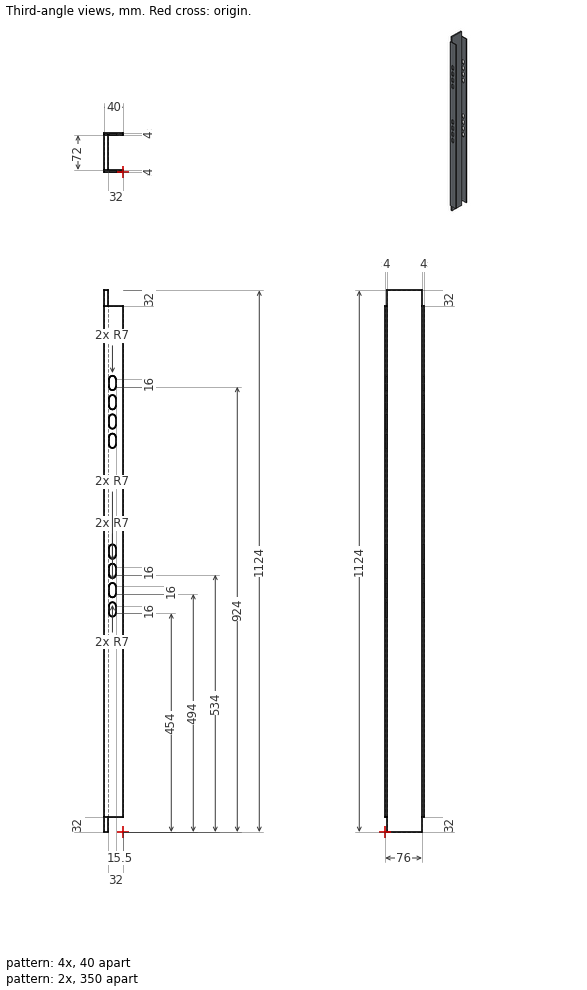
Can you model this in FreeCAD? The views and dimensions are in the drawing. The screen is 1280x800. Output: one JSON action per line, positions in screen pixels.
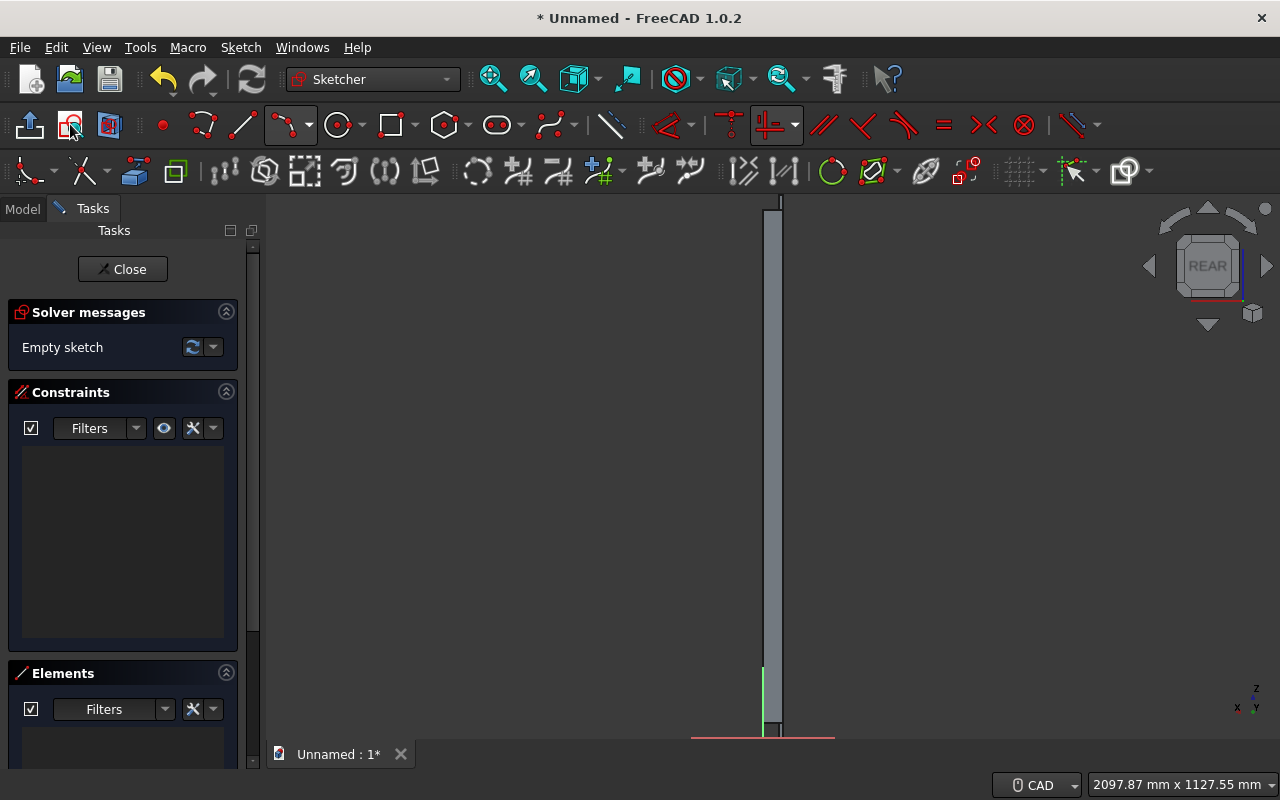
{"action": "scroll", "coordinate": [778, 278], "scroll_direction": "up", "scroll_amount": 15}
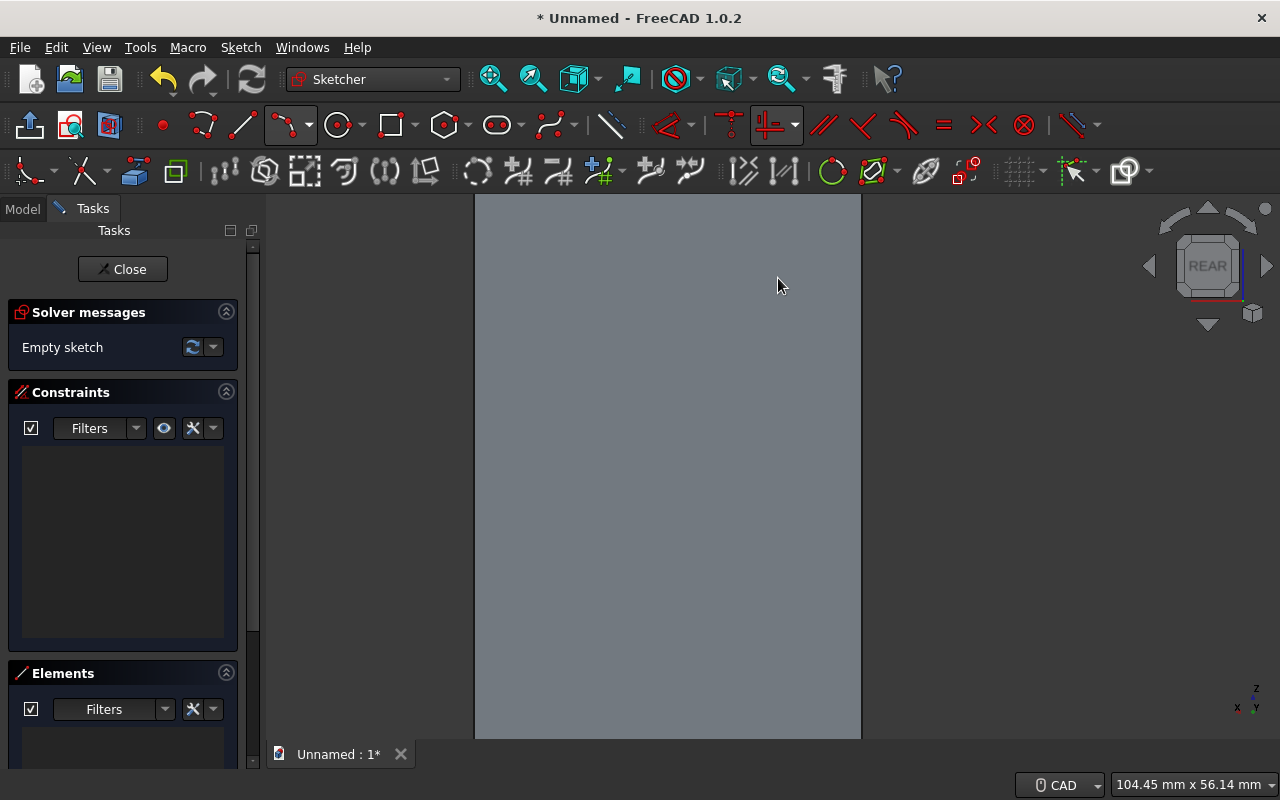
{"action": "left_click", "coordinate": [498, 126]}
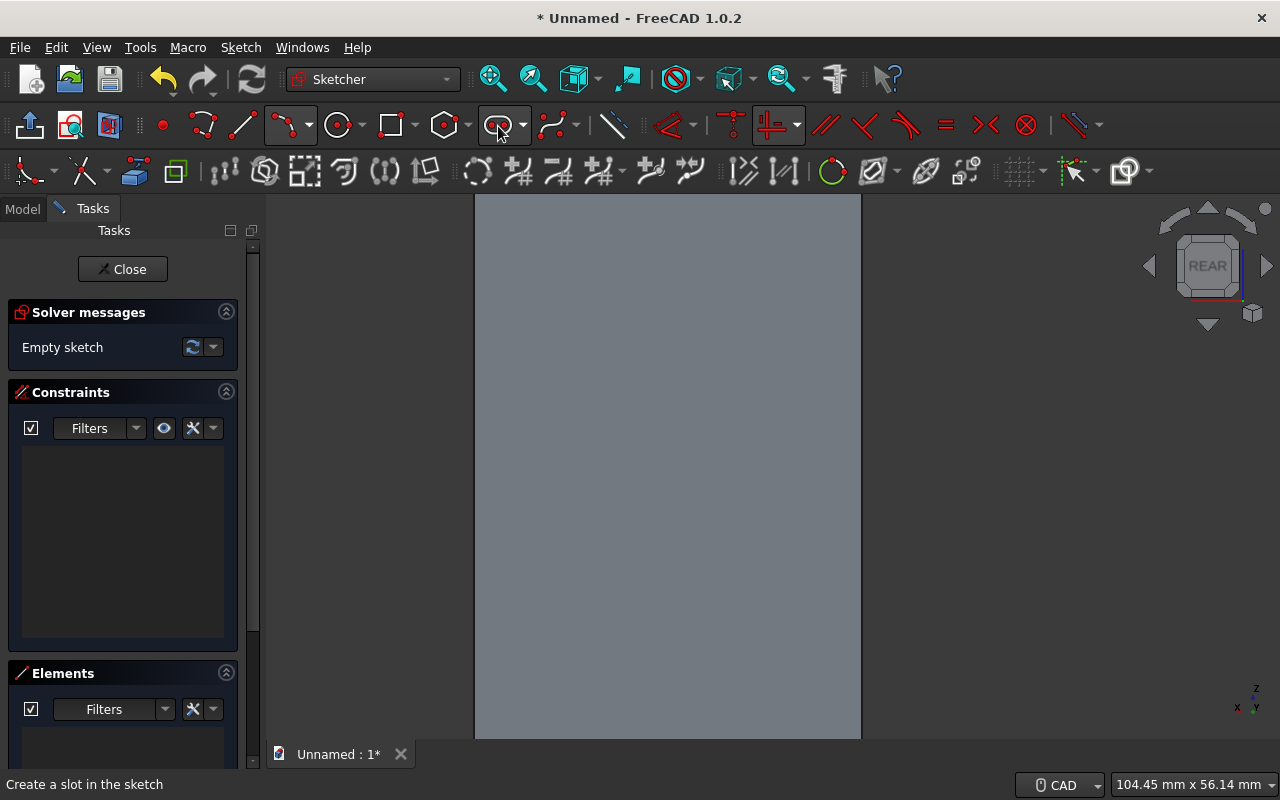
{"action": "left_click", "coordinate": [692, 547]}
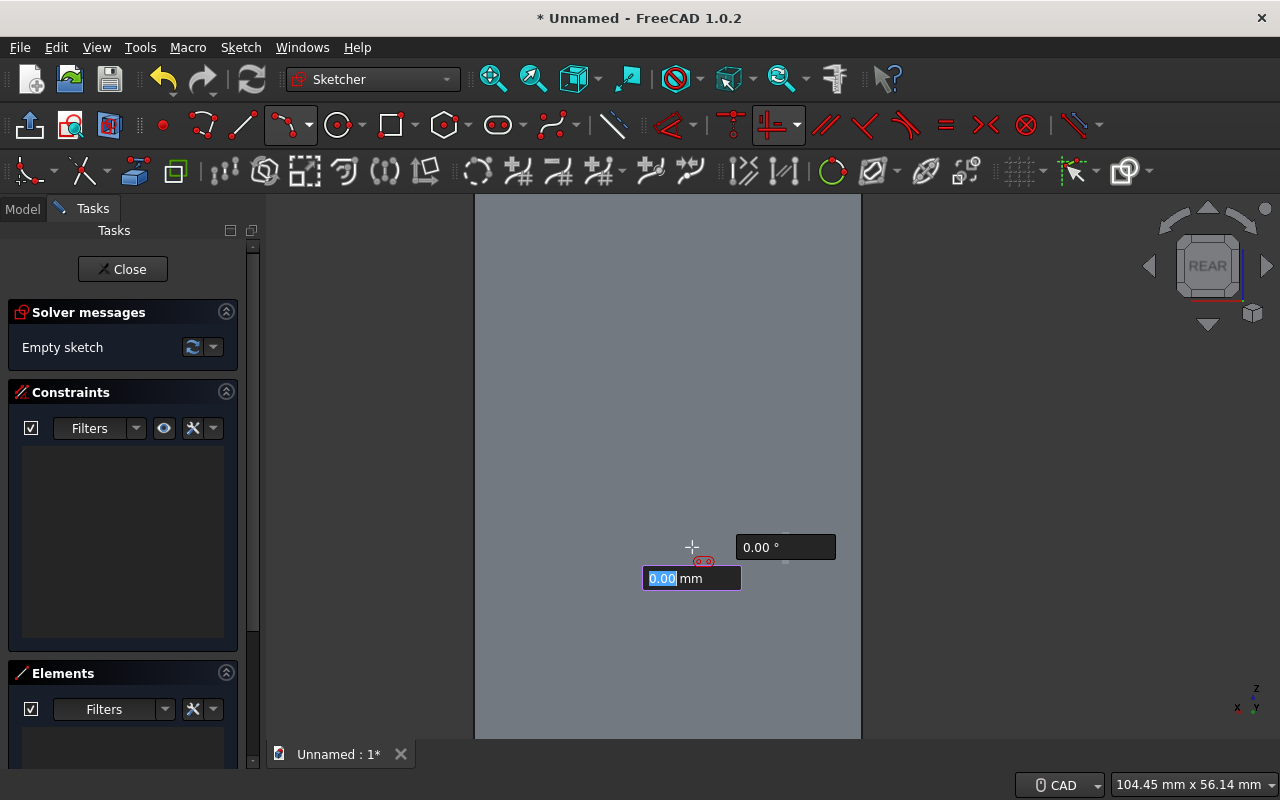
{"action": "left_click", "coordinate": [692, 391]}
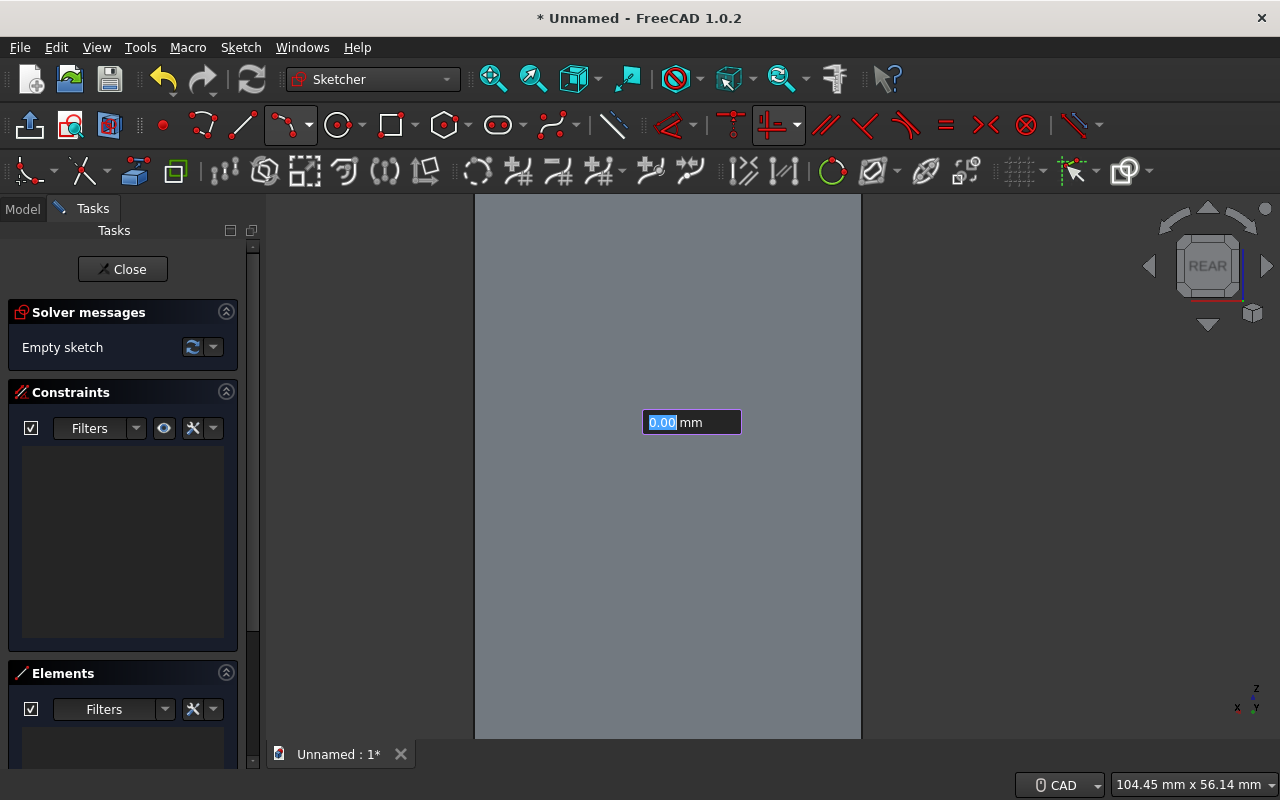
{"action": "left_click", "coordinate": [760, 469]}
{"action": "key", "text": "Escape"}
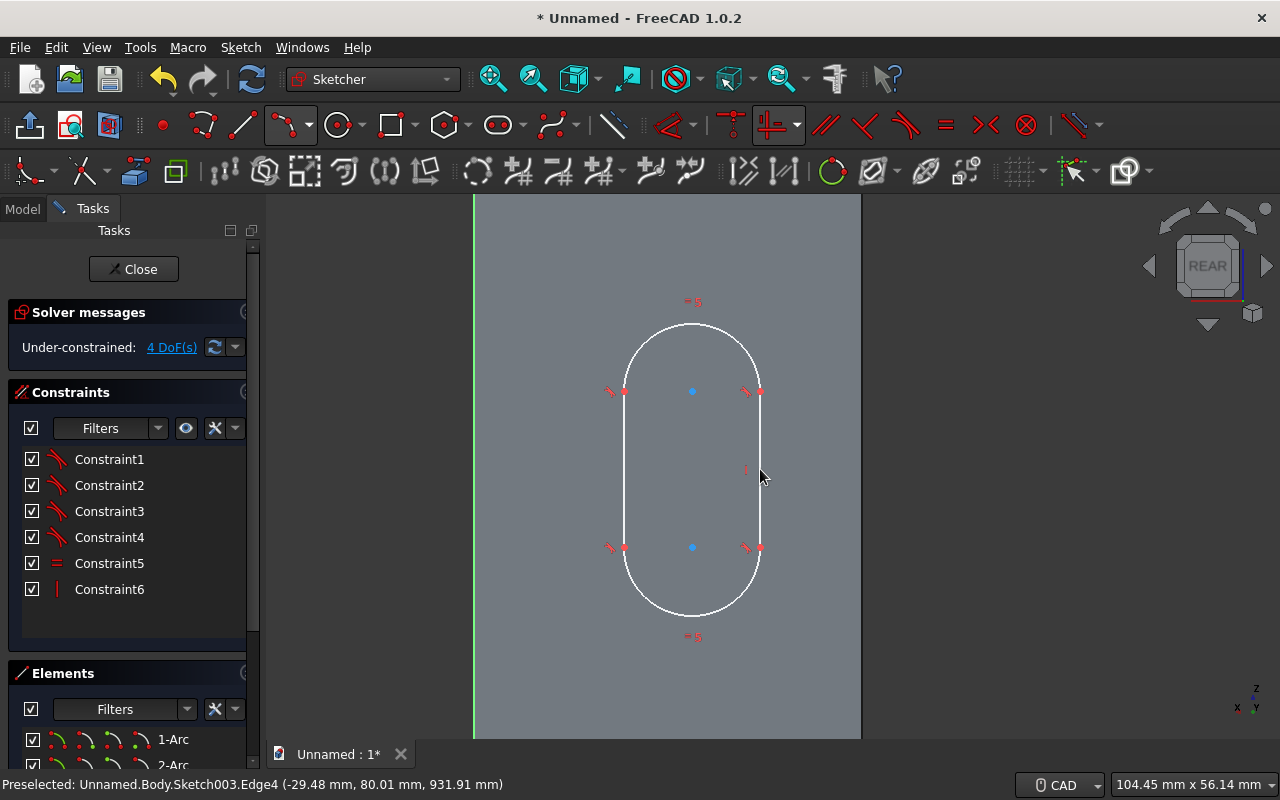
{"action": "left_click", "coordinate": [668, 126]}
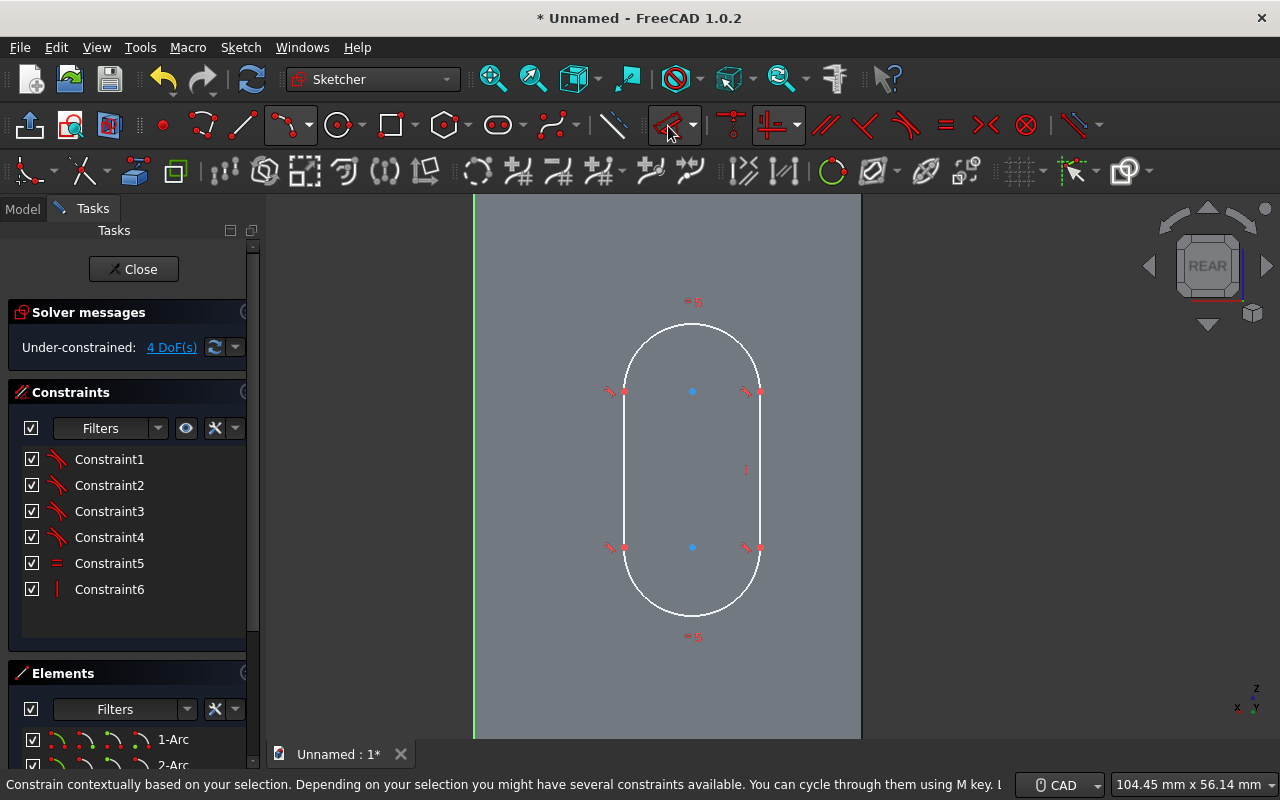
{"action": "left_click", "coordinate": [652, 603]}
{"action": "left_click", "coordinate": [633, 629]}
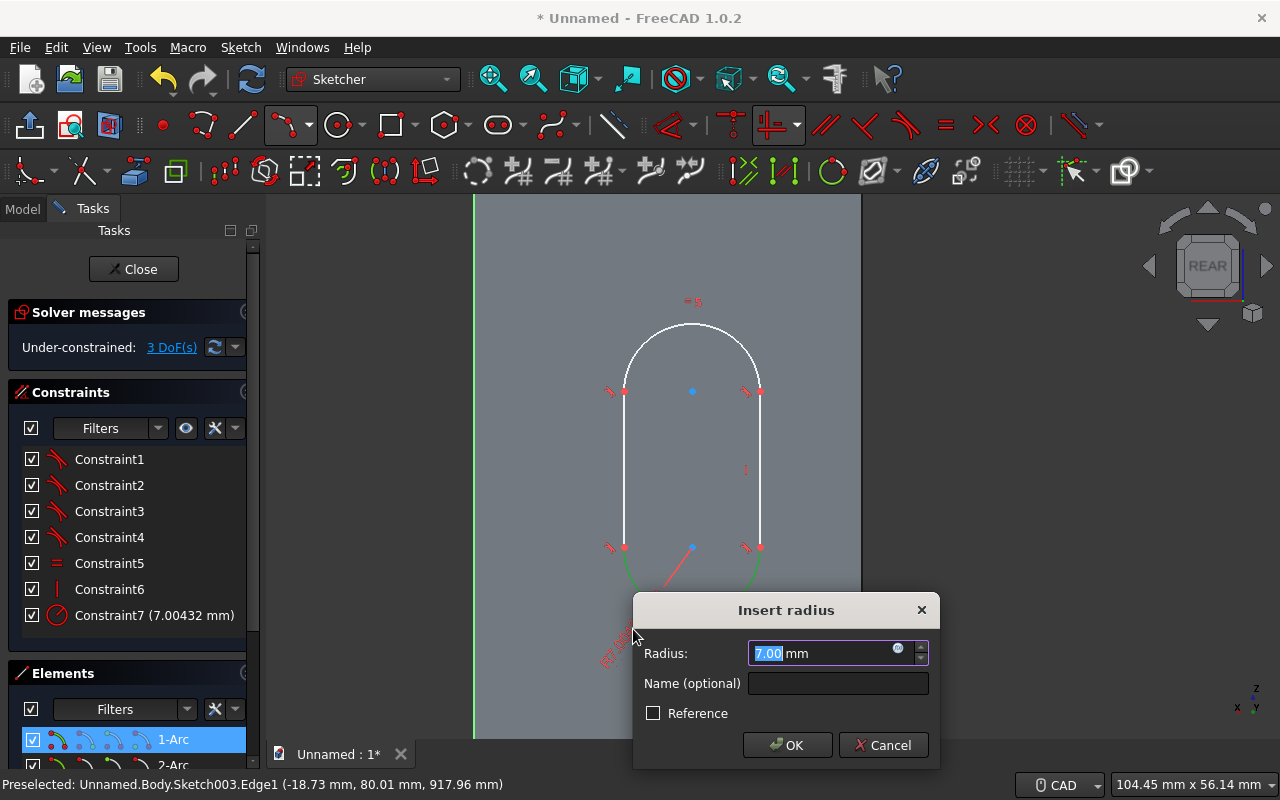
{"action": "type", "text": "7"}
{"action": "key", "text": "Return"}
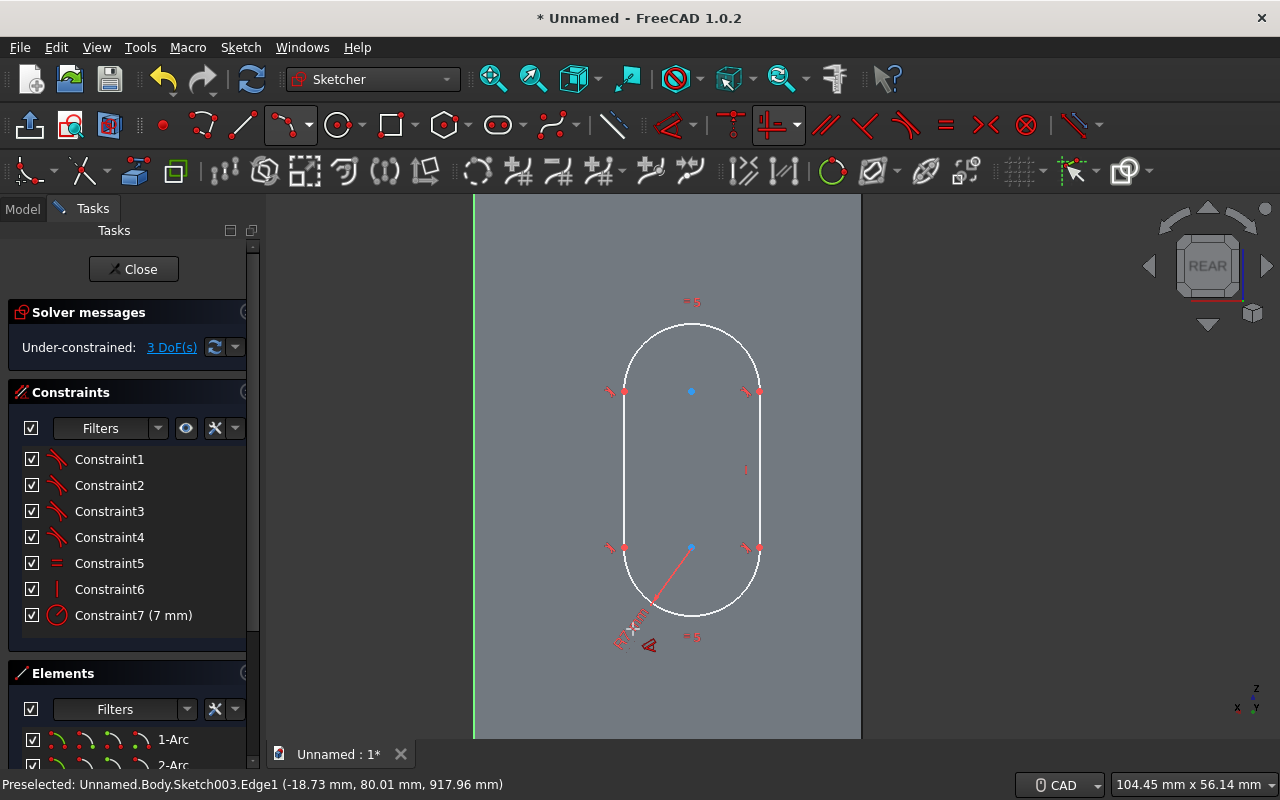
{"action": "left_click", "coordinate": [624, 501]}
{"action": "left_click", "coordinate": [590, 470]}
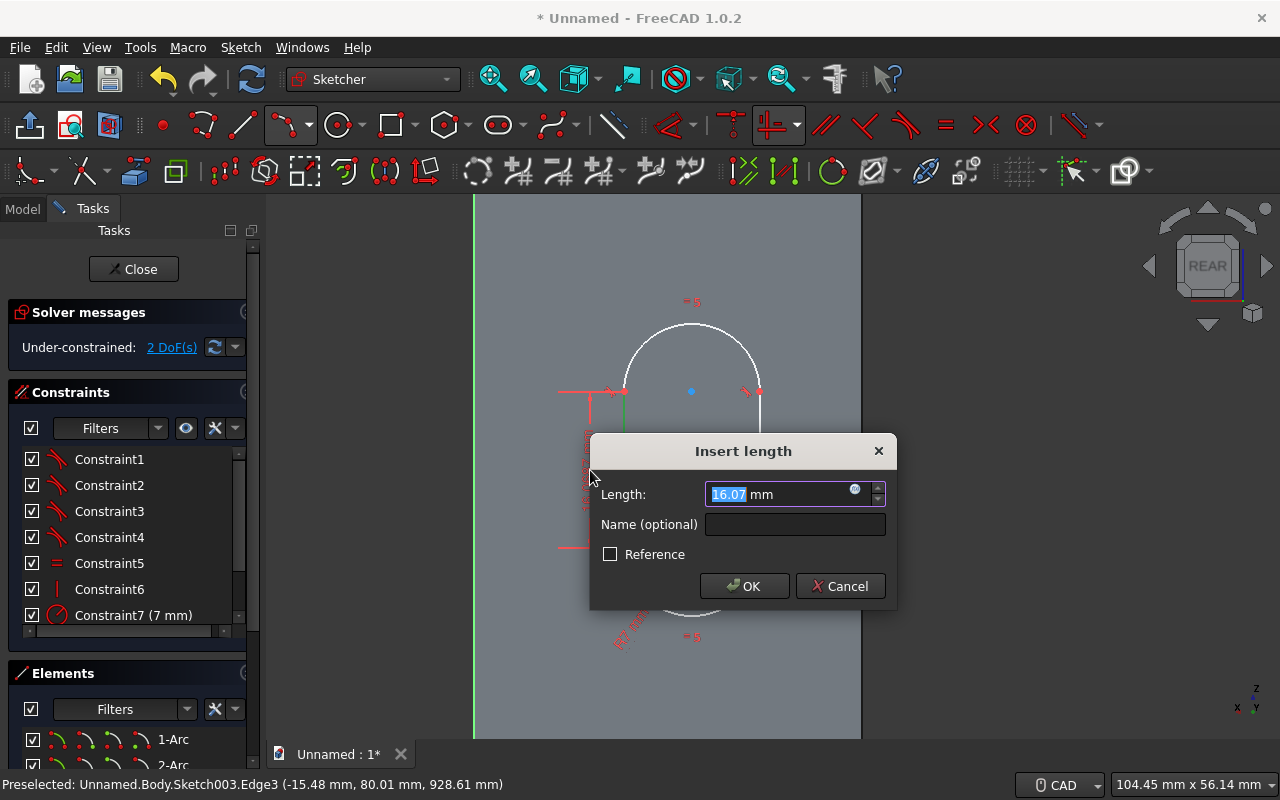
{"action": "type", "text": "16"}
{"action": "key", "text": "Return"}